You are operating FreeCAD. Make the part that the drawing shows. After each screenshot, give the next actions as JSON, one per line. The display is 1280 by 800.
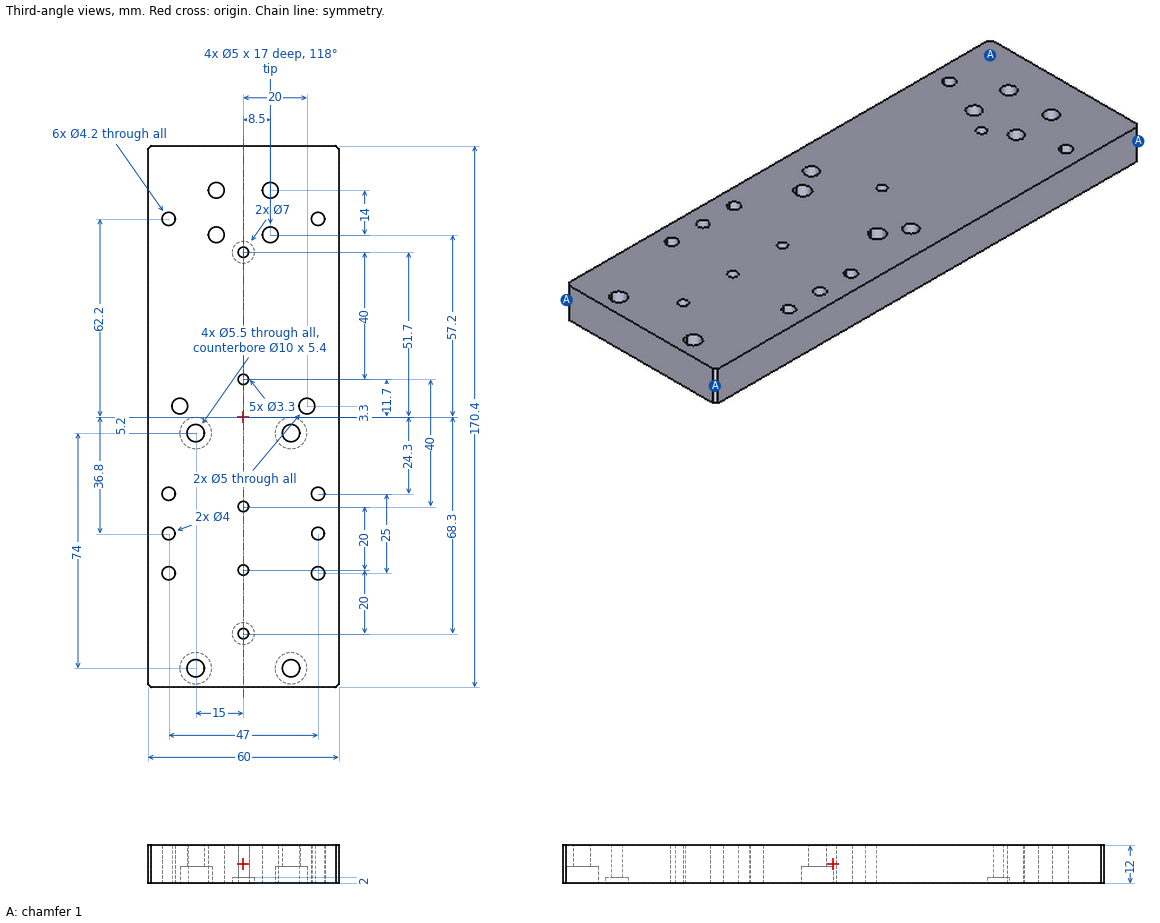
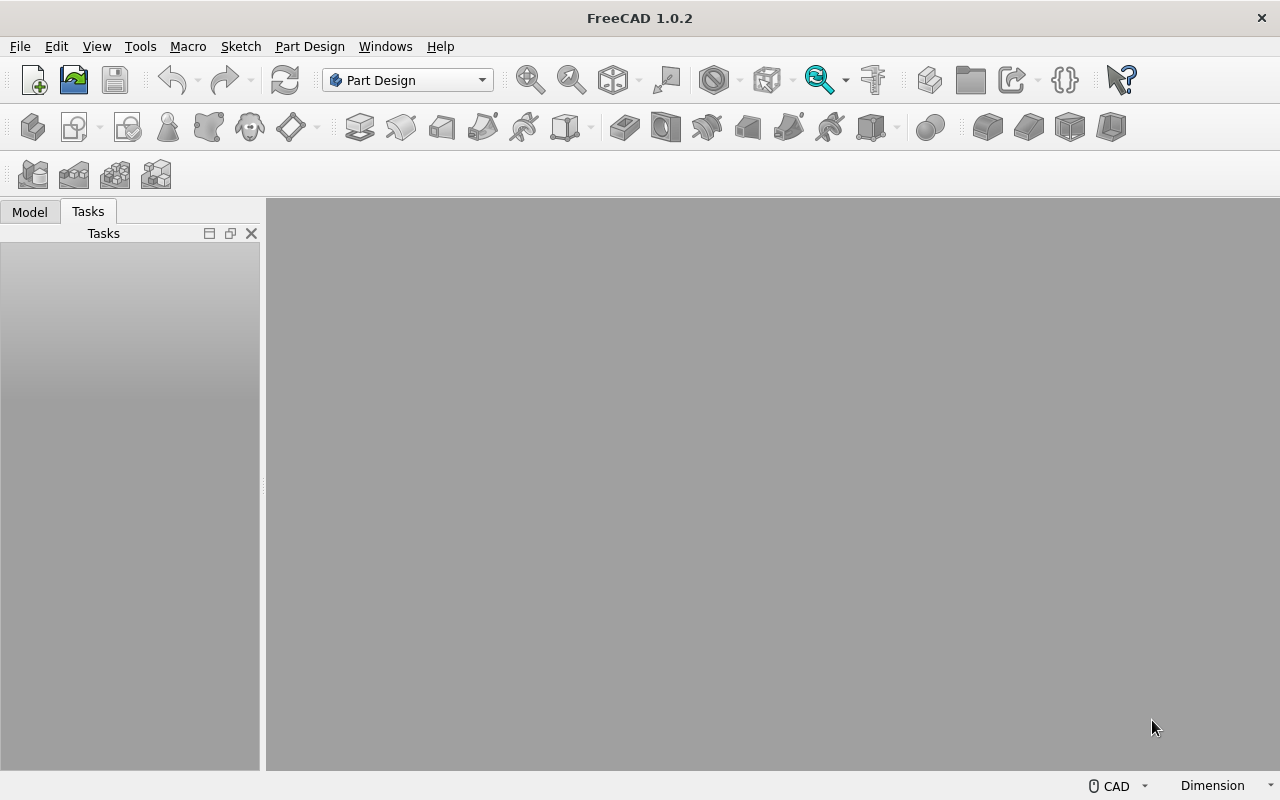
{"action": "left_click", "coordinate": [33, 80]}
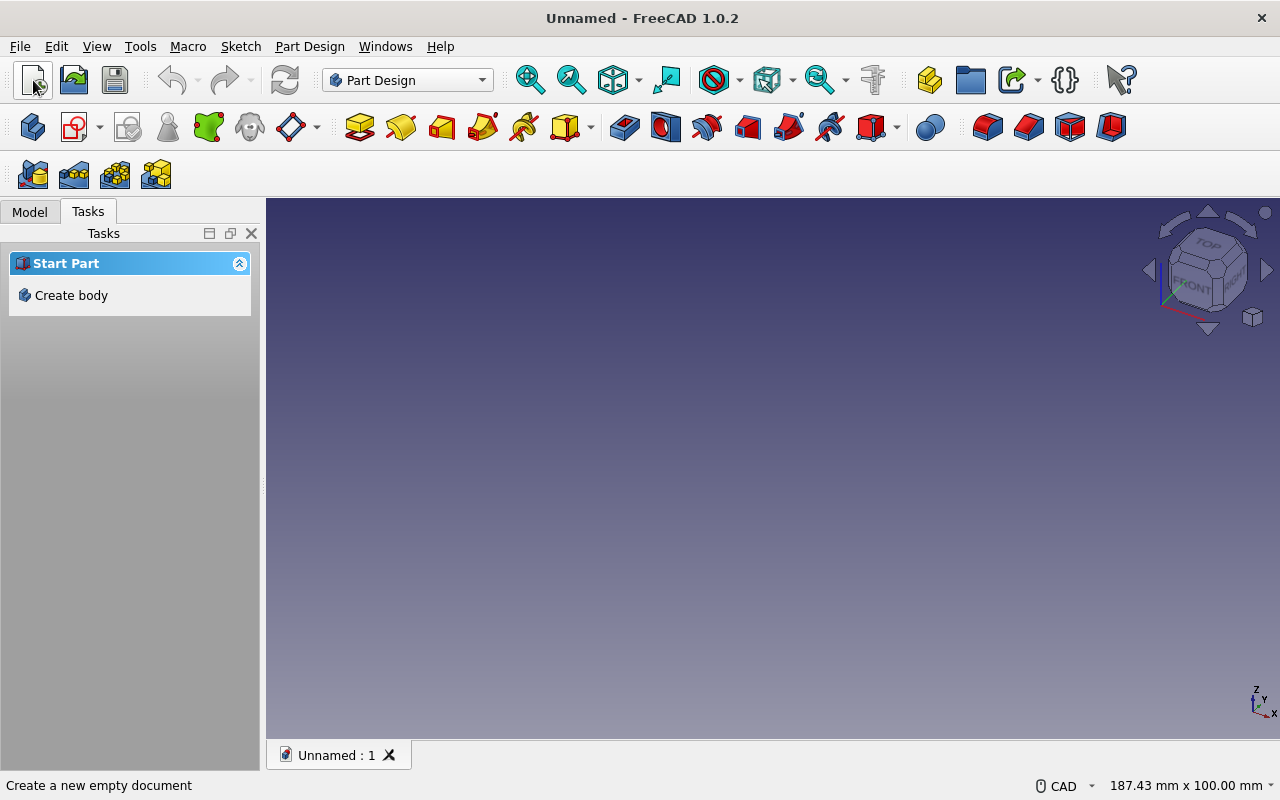
{"action": "left_click", "coordinate": [74, 128]}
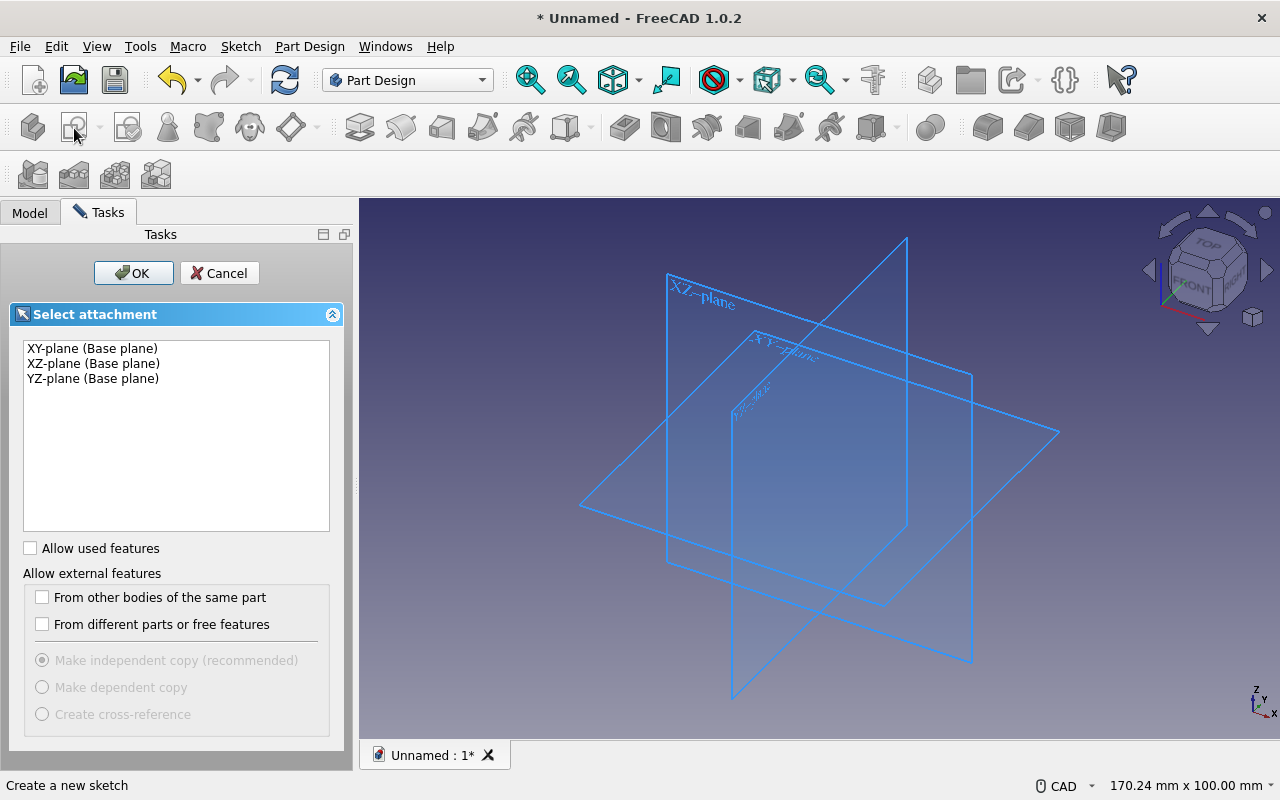
{"action": "left_click", "coordinate": [84, 348]}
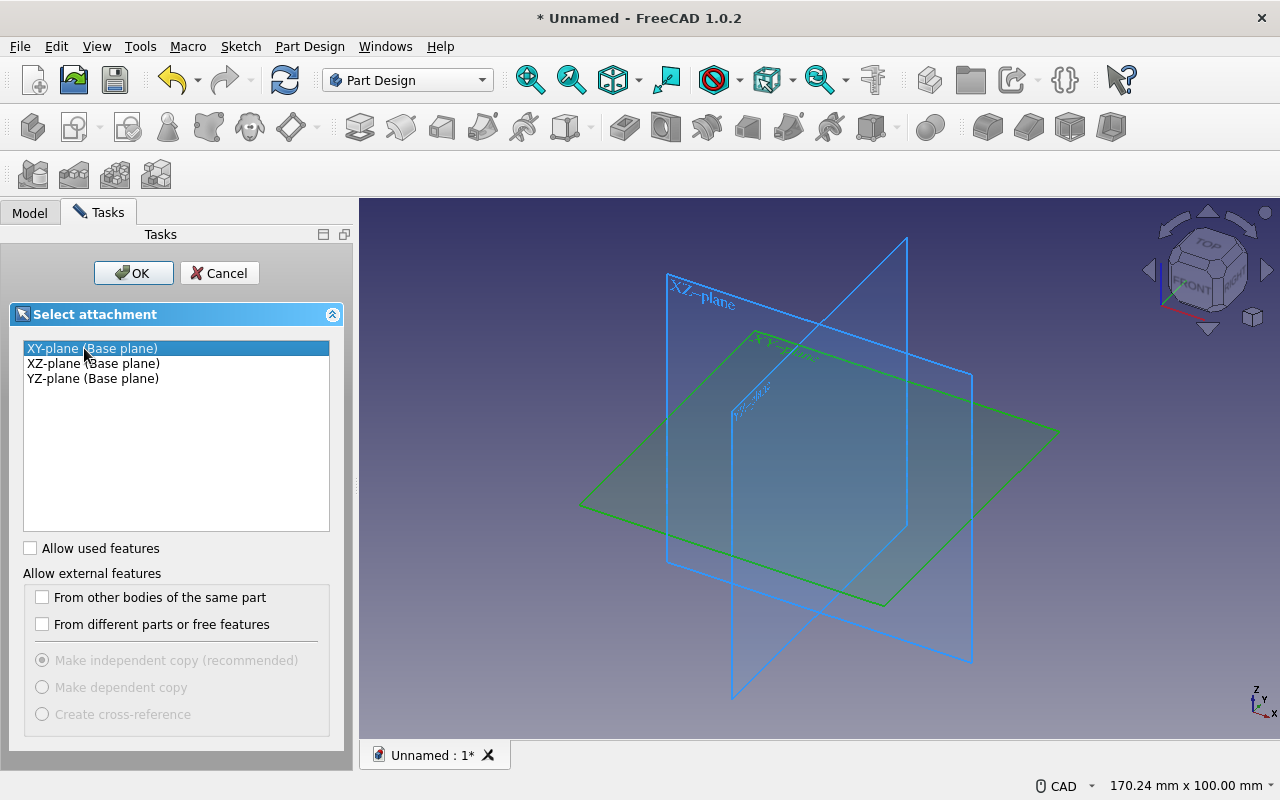
{"action": "left_click", "coordinate": [134, 273]}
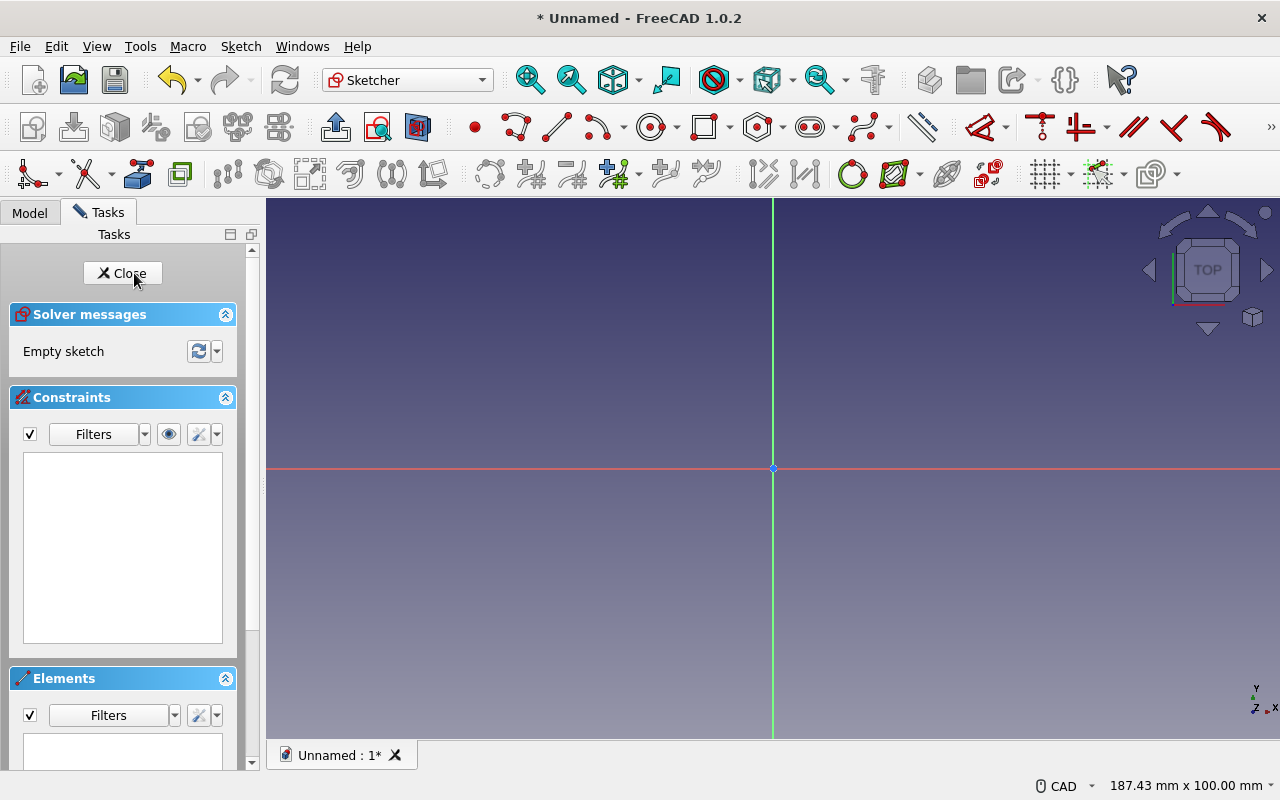
{"action": "scroll", "coordinate": [665, 469], "scroll_direction": "down", "scroll_amount": 5}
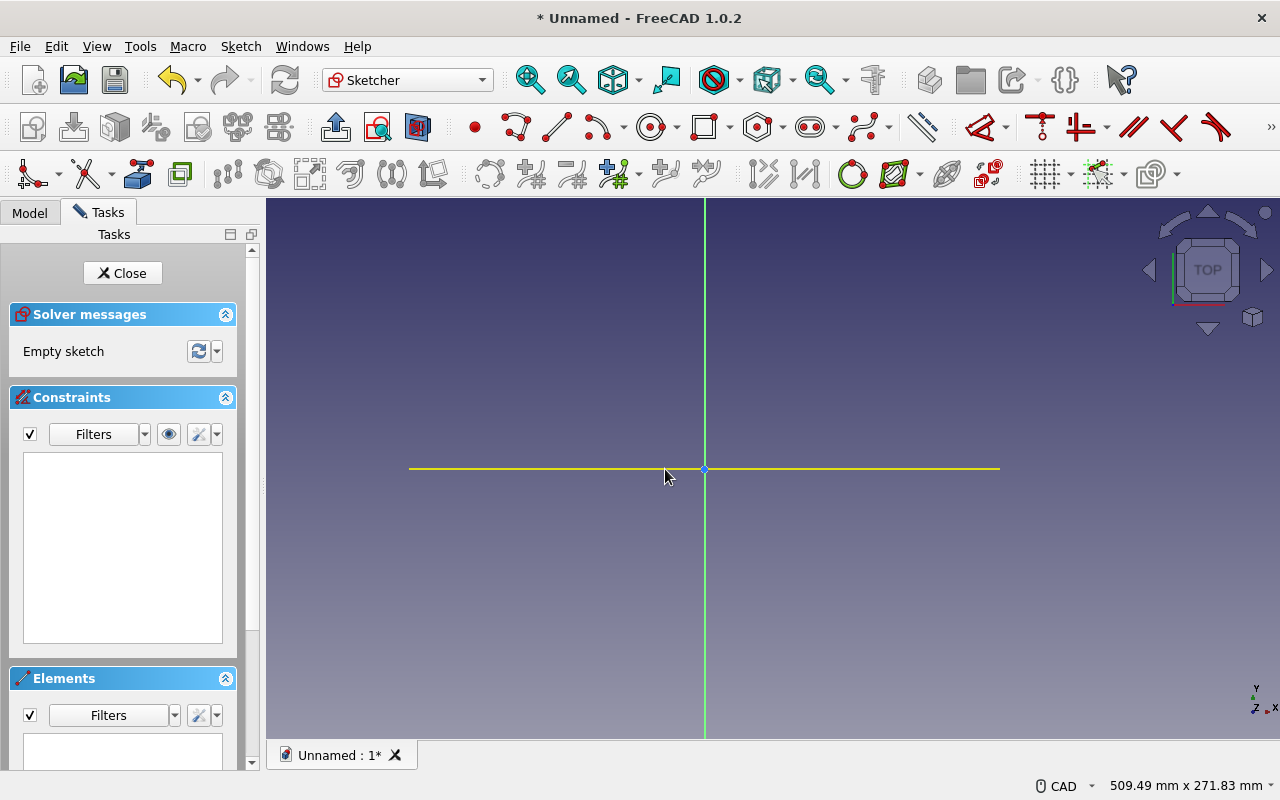
{"action": "key", "text": "g v"}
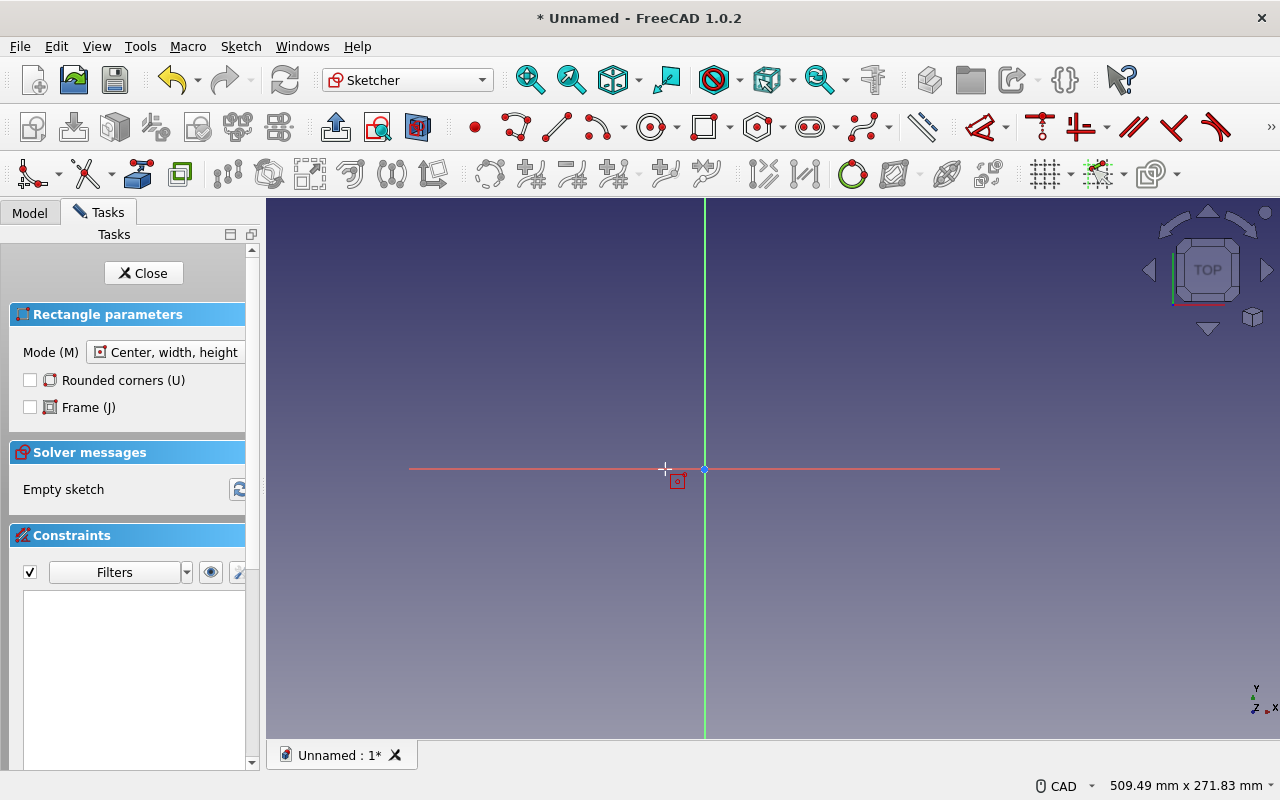
{"action": "left_click", "coordinate": [705, 469]}
{"action": "left_click", "coordinate": [765, 300]}
{"action": "key", "text": "Escape"}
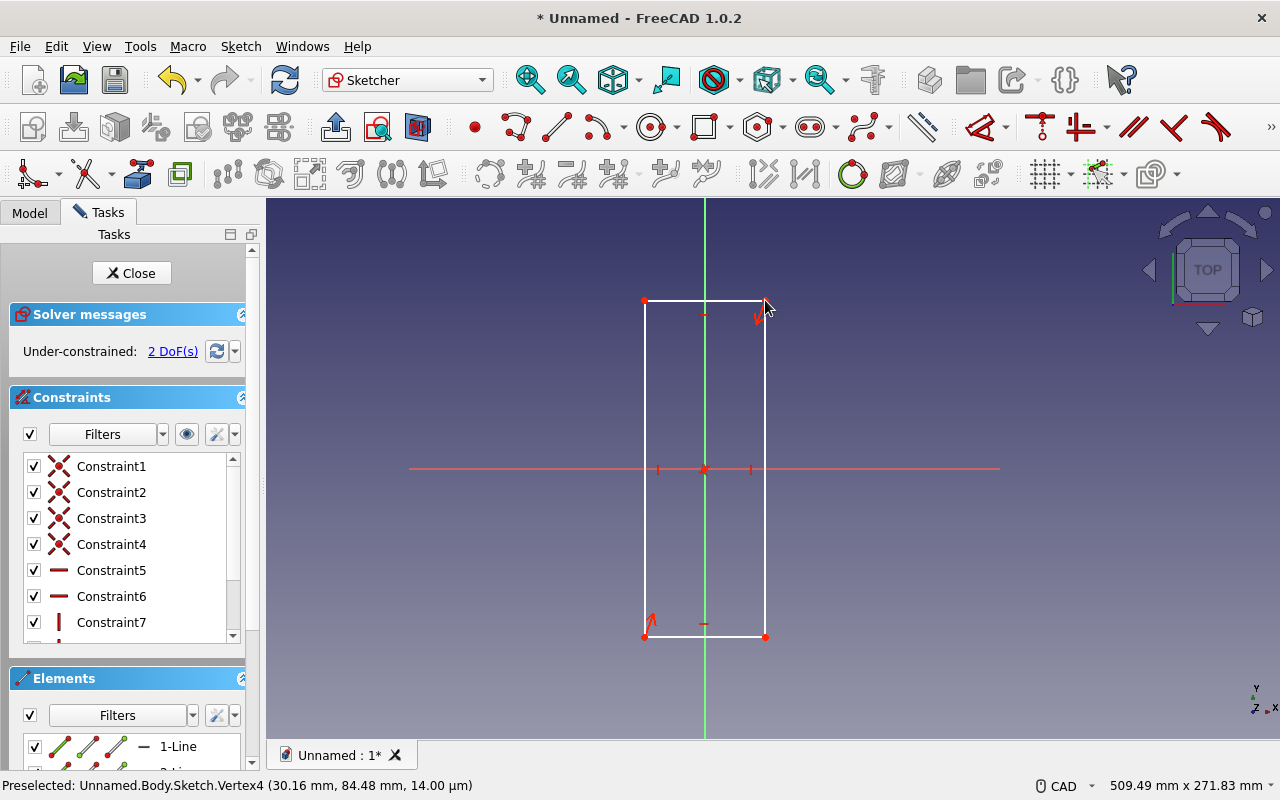
{"action": "left_click", "coordinate": [980, 128]}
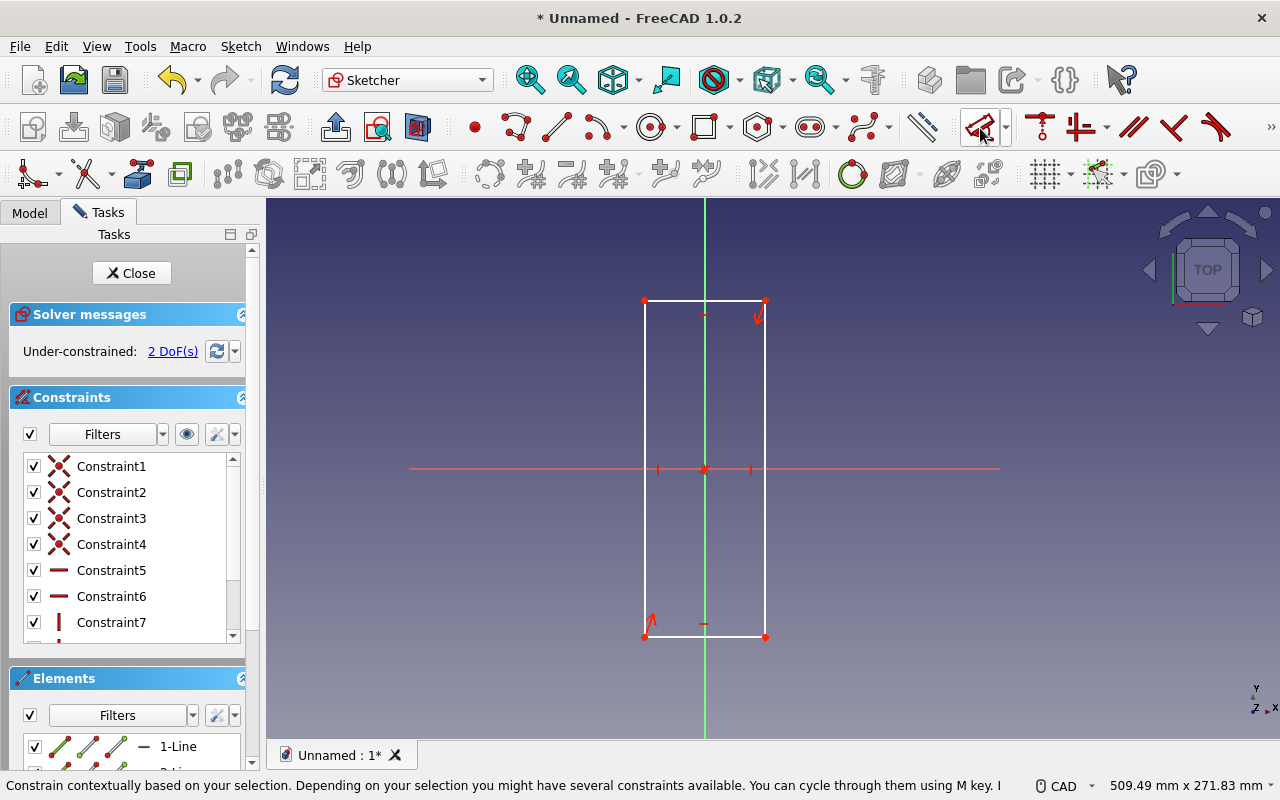
{"action": "left_click", "coordinate": [681, 637]}
{"action": "left_click", "coordinate": [677, 671]}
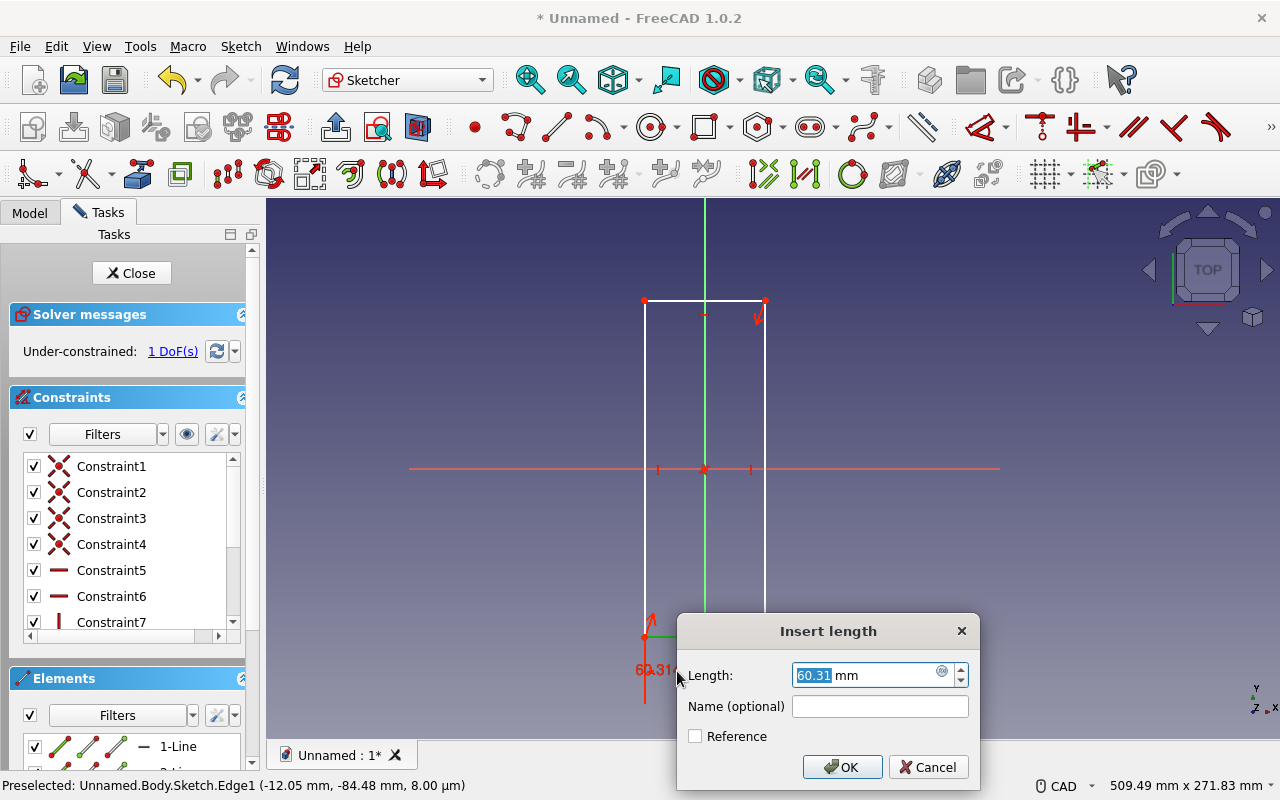
{"action": "type", "text": "60"}
{"action": "key", "text": "Return"}